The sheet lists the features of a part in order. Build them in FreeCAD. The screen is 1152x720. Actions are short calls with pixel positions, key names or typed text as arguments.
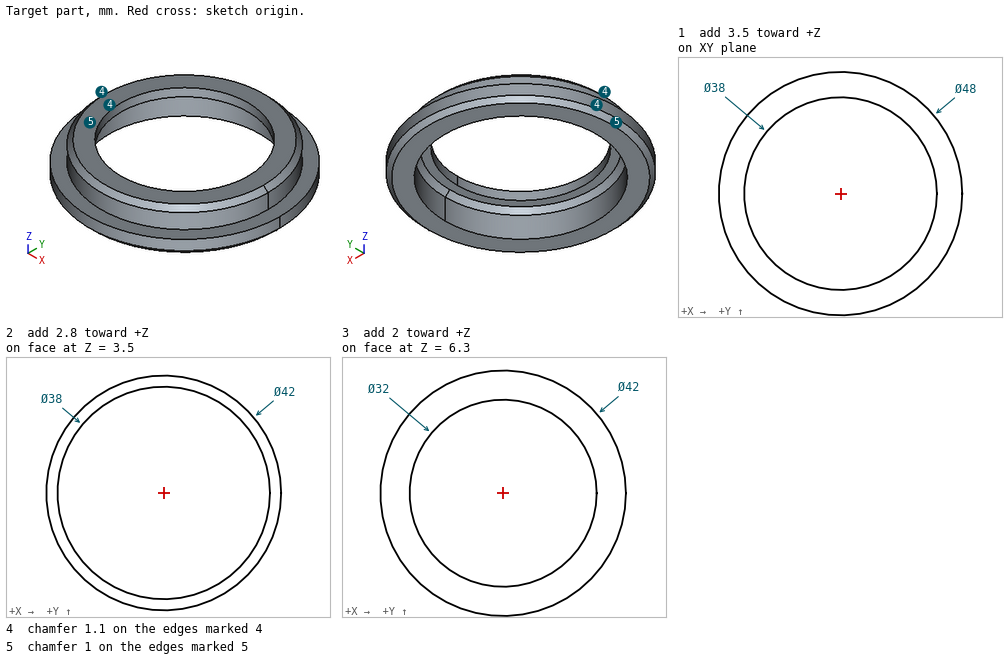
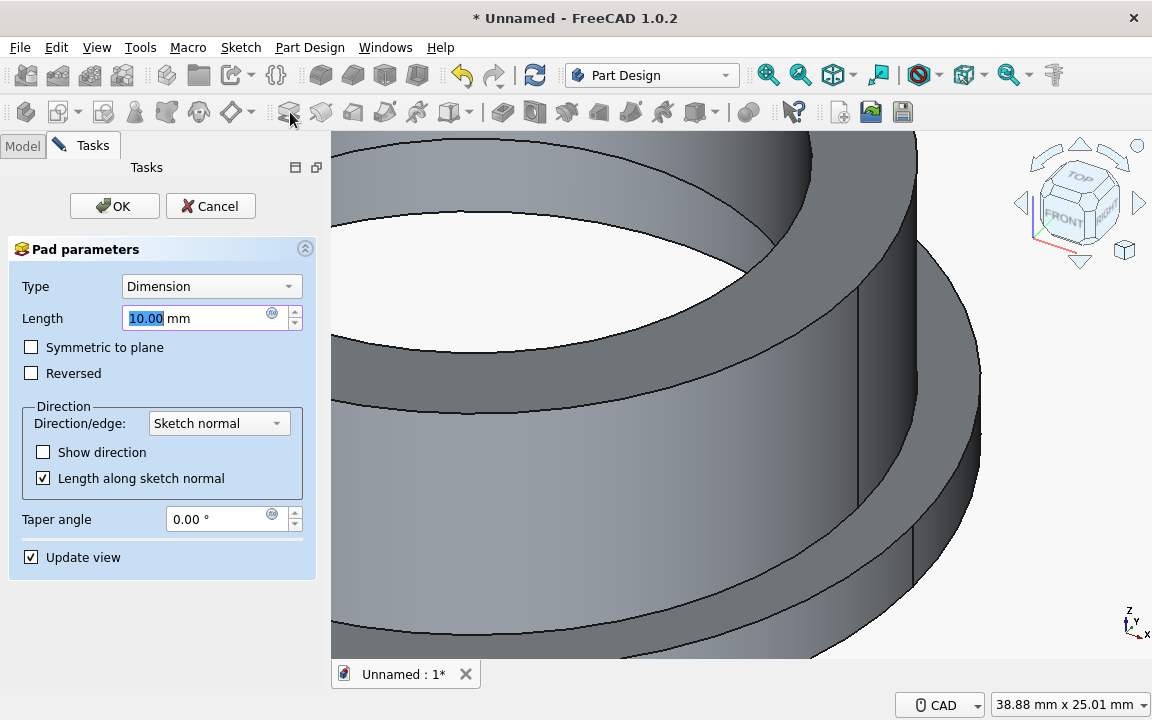
text(2)
key(Tab)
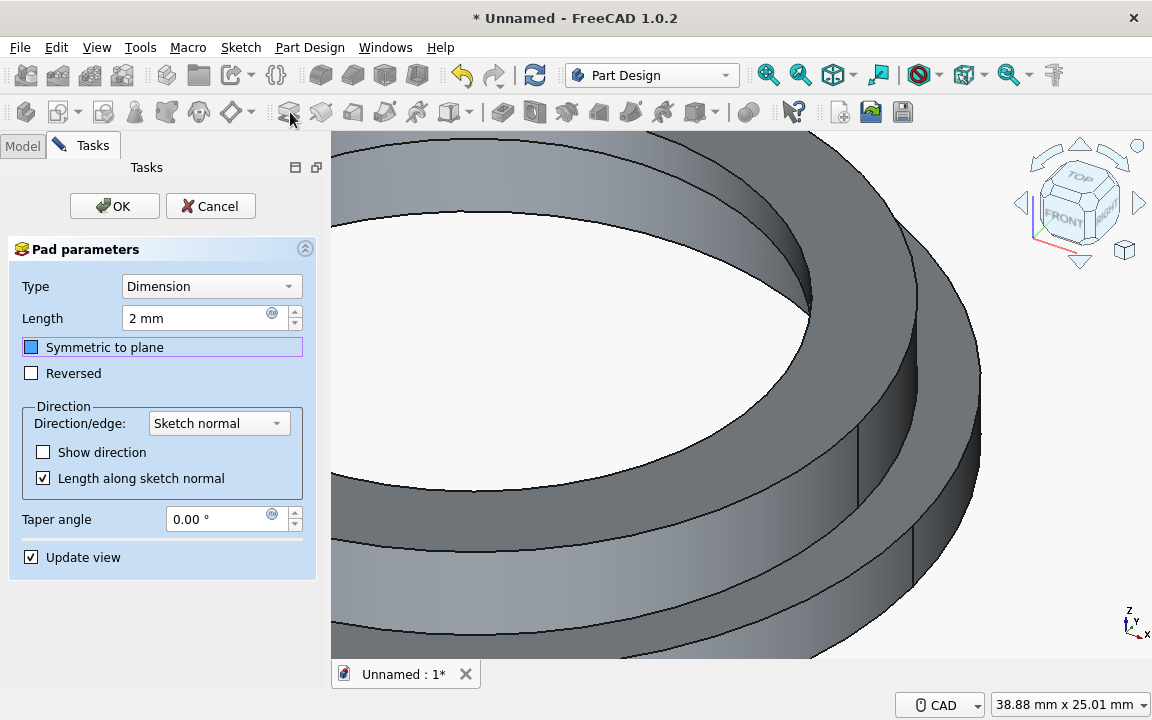
click(115, 206)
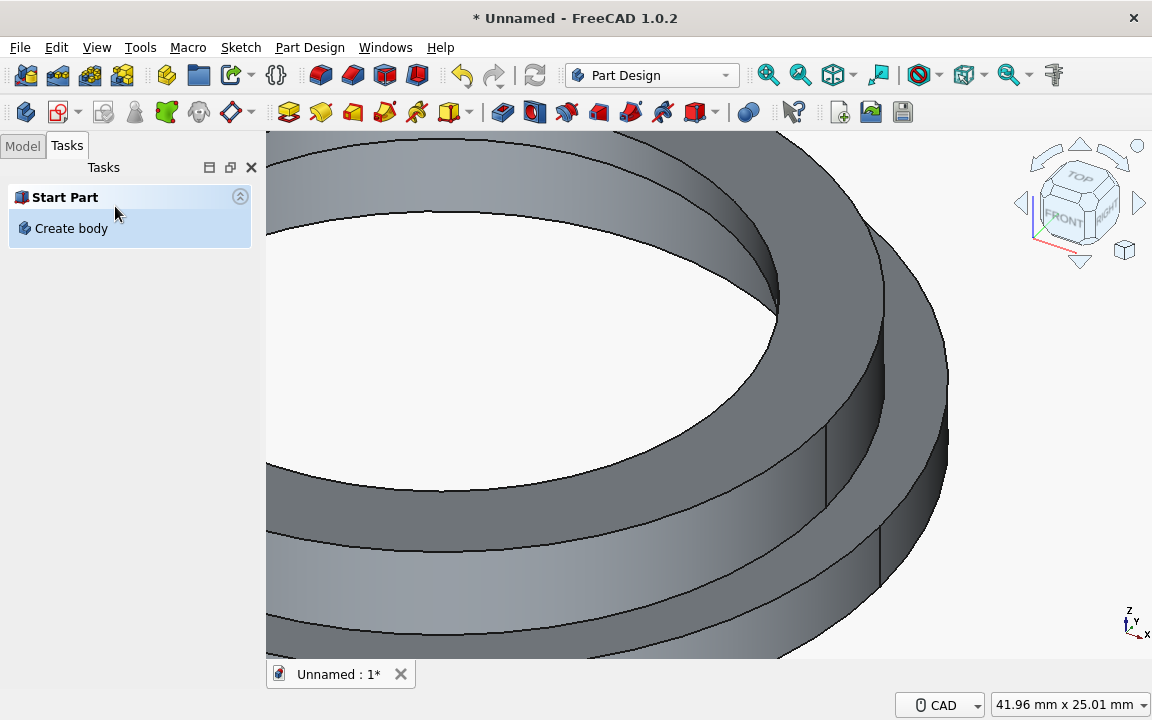
click(770, 76)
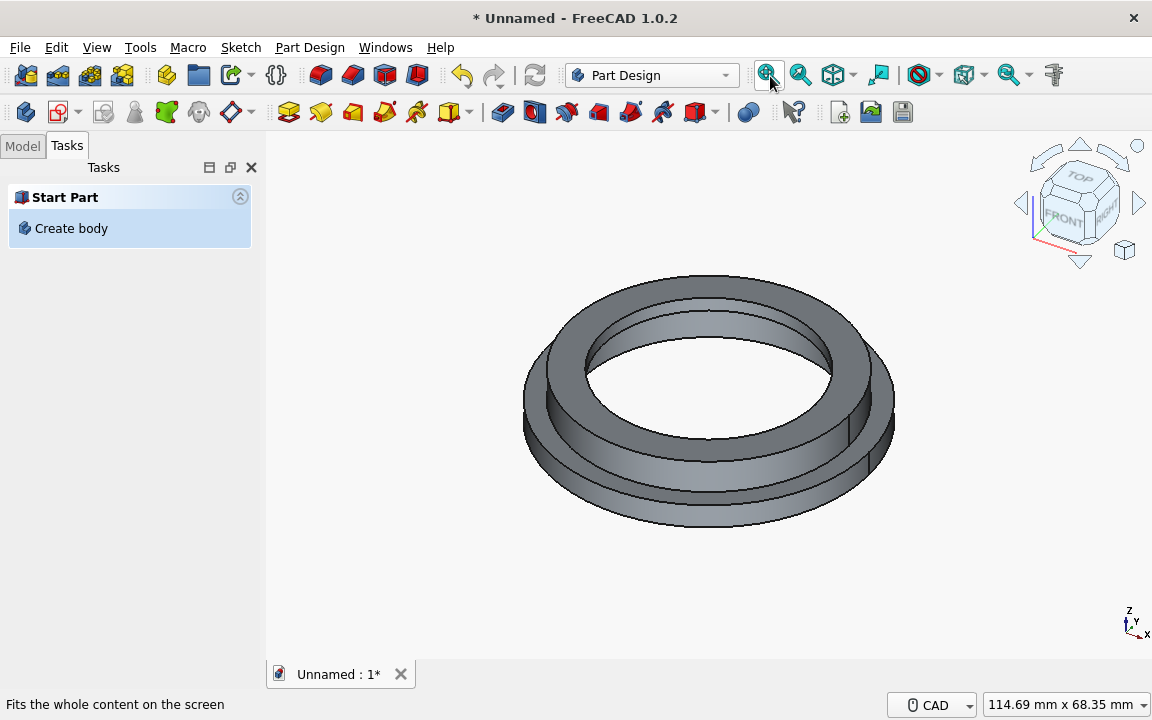
click(548, 377)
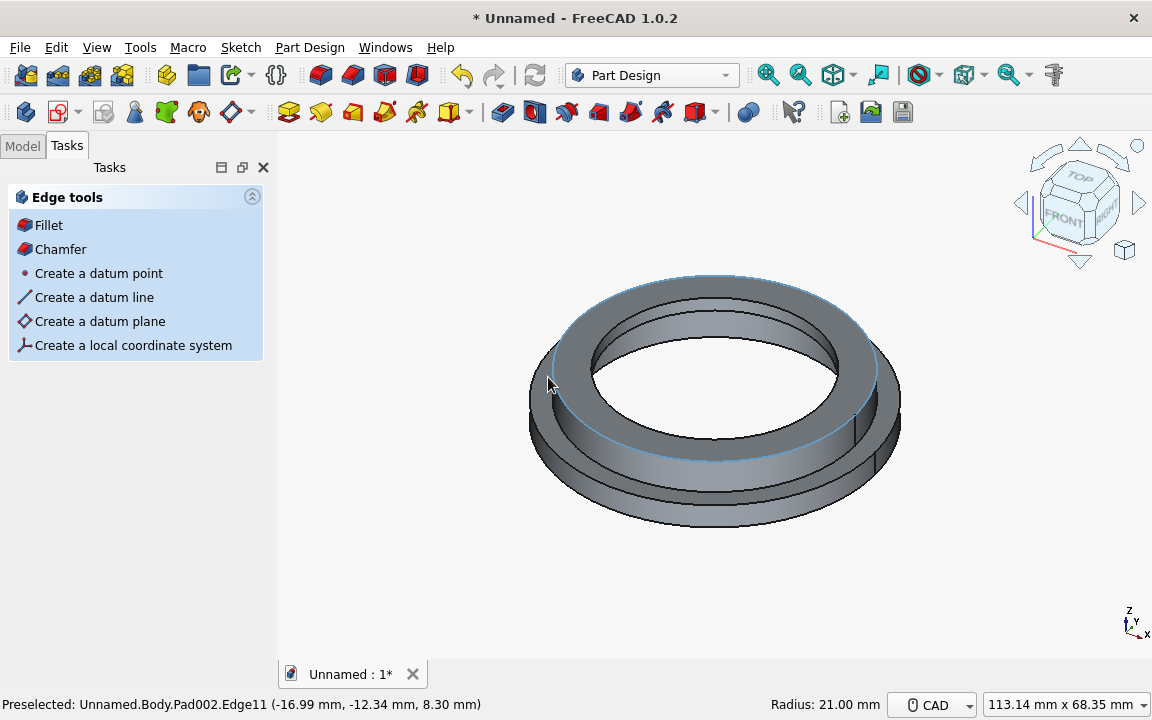
key(0)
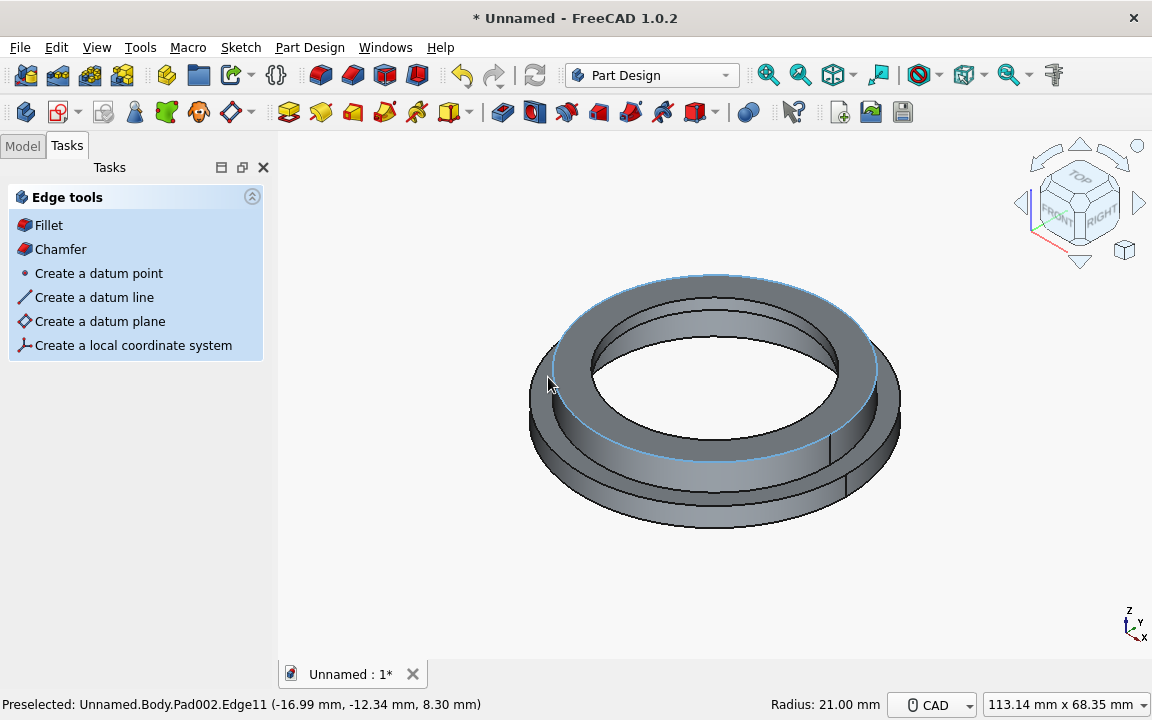
key(2)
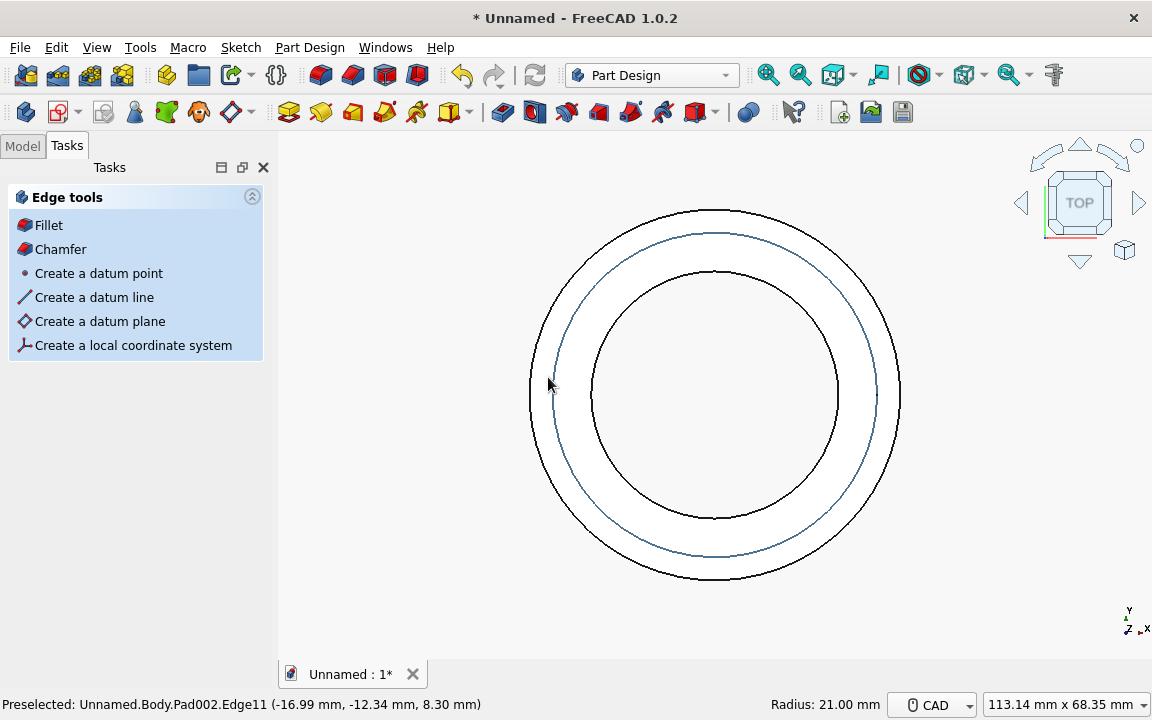
key(1)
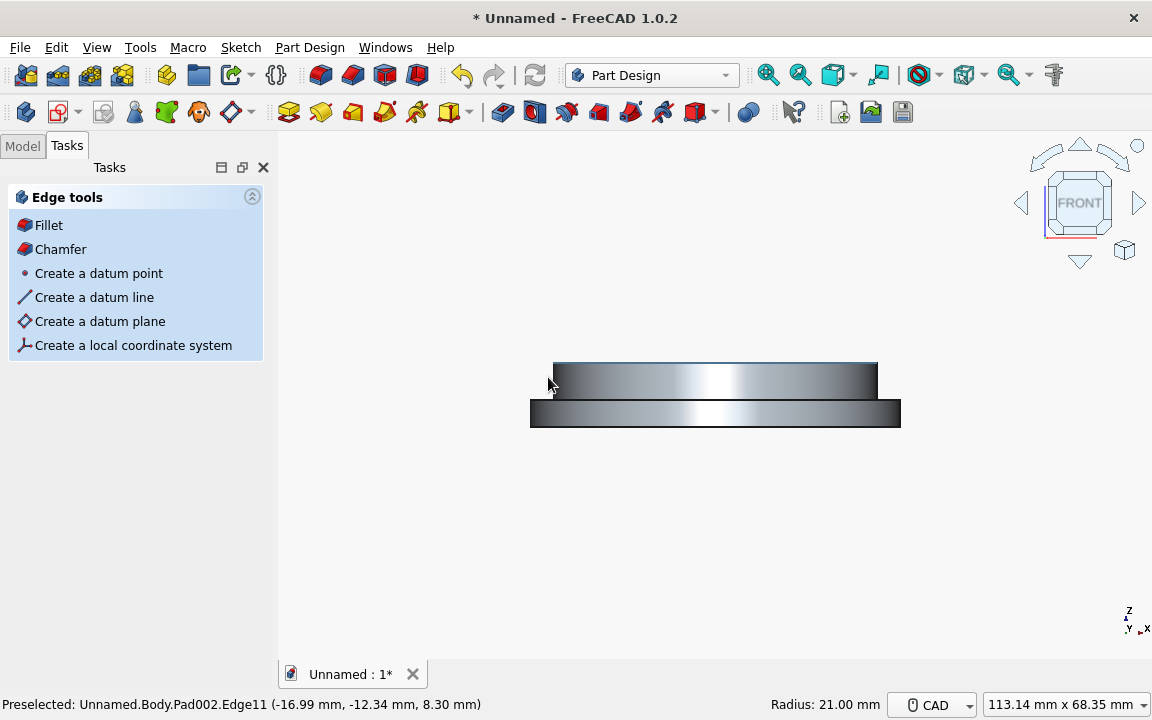
click(770, 76)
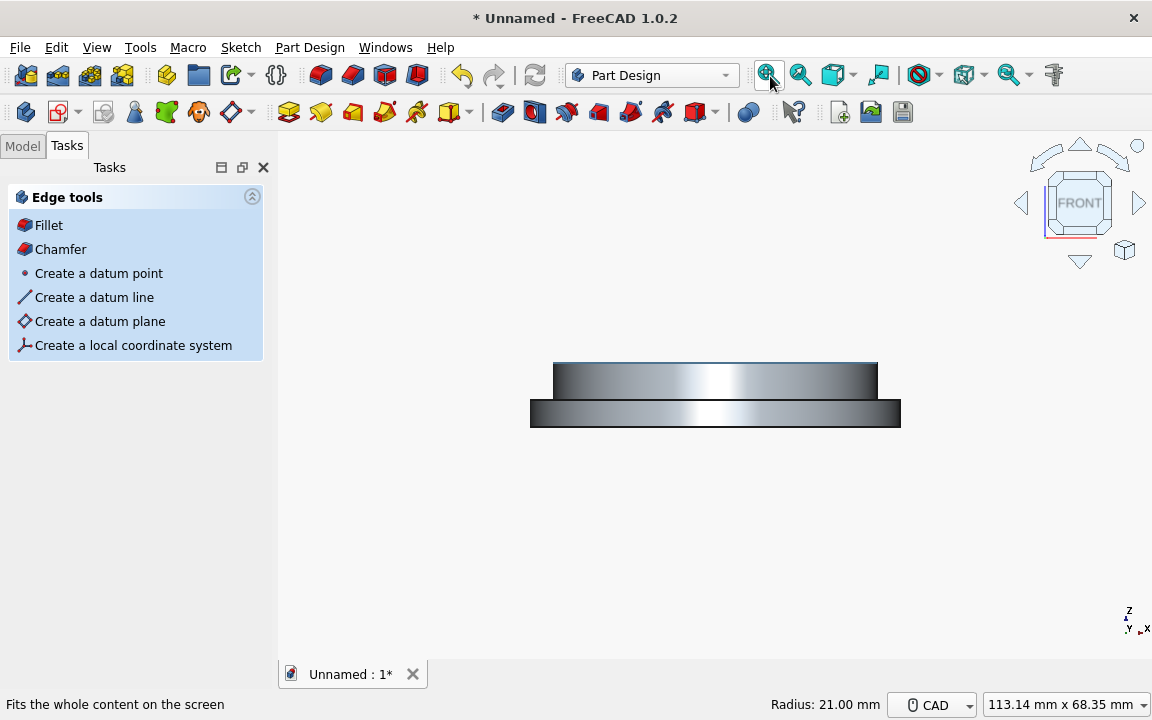
key(3)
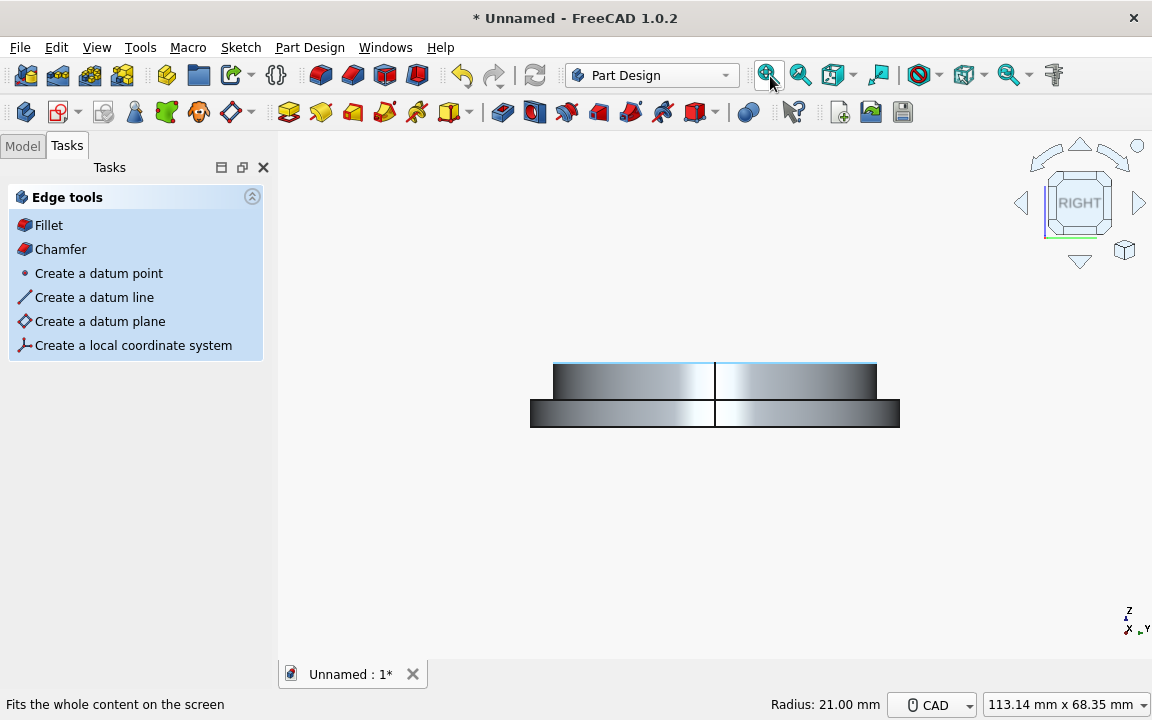
click(770, 76)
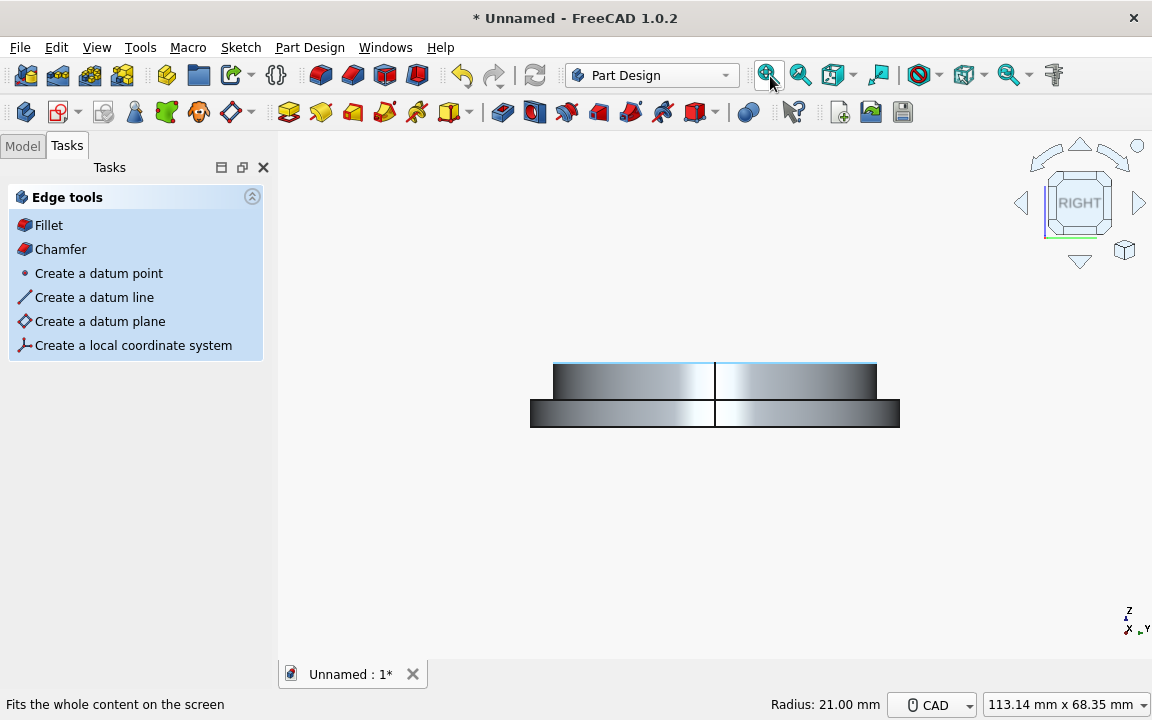
key(5)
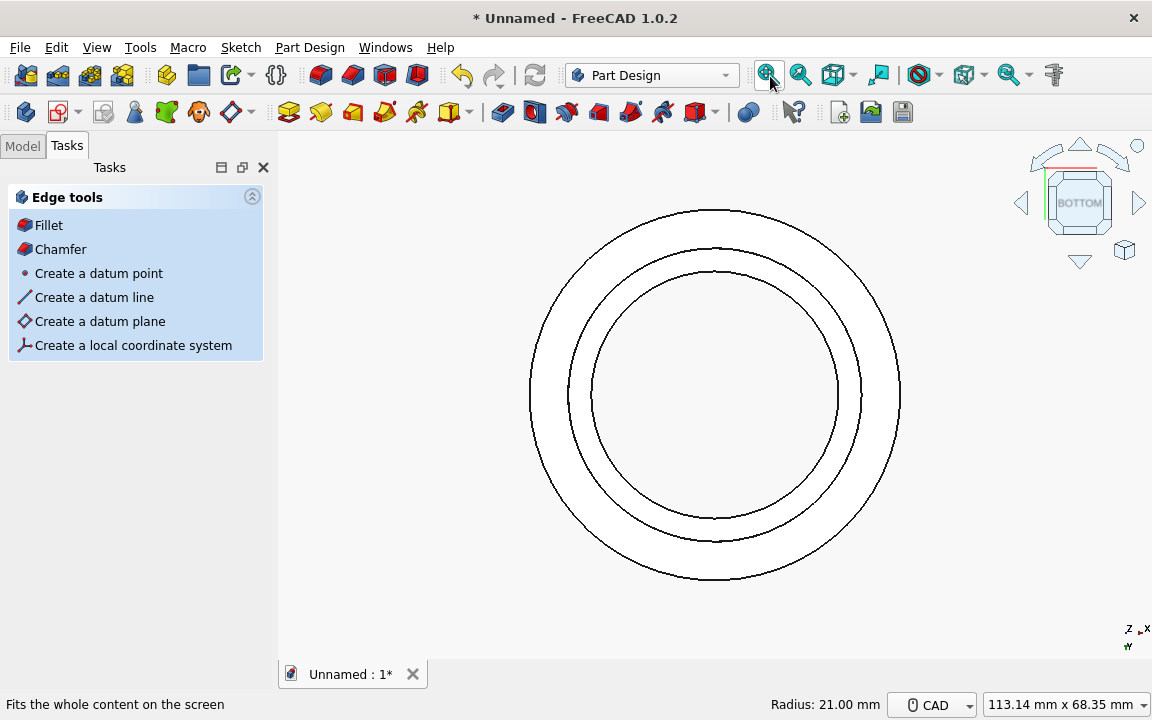
key(4)